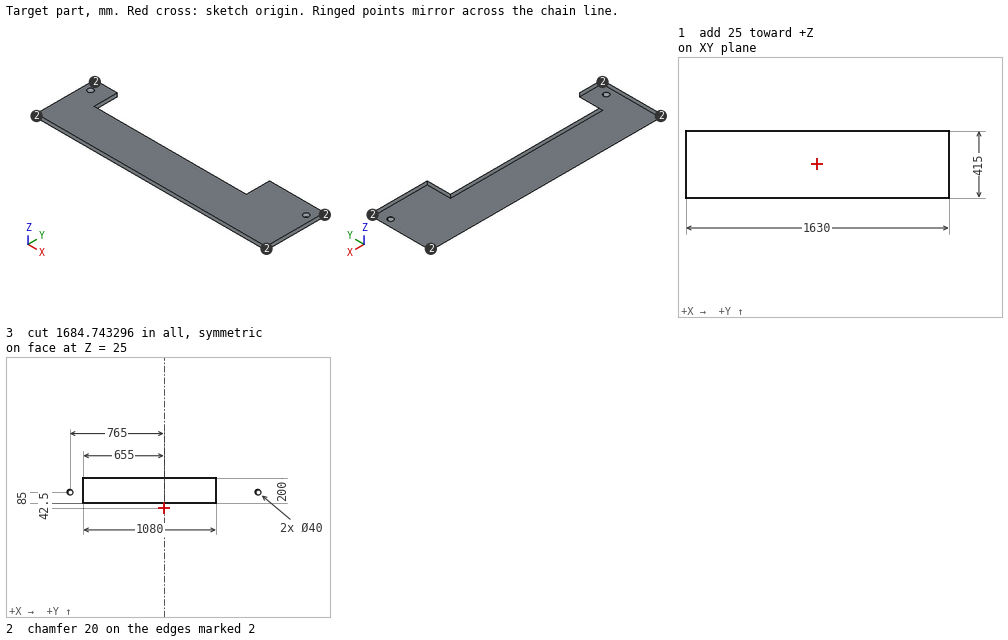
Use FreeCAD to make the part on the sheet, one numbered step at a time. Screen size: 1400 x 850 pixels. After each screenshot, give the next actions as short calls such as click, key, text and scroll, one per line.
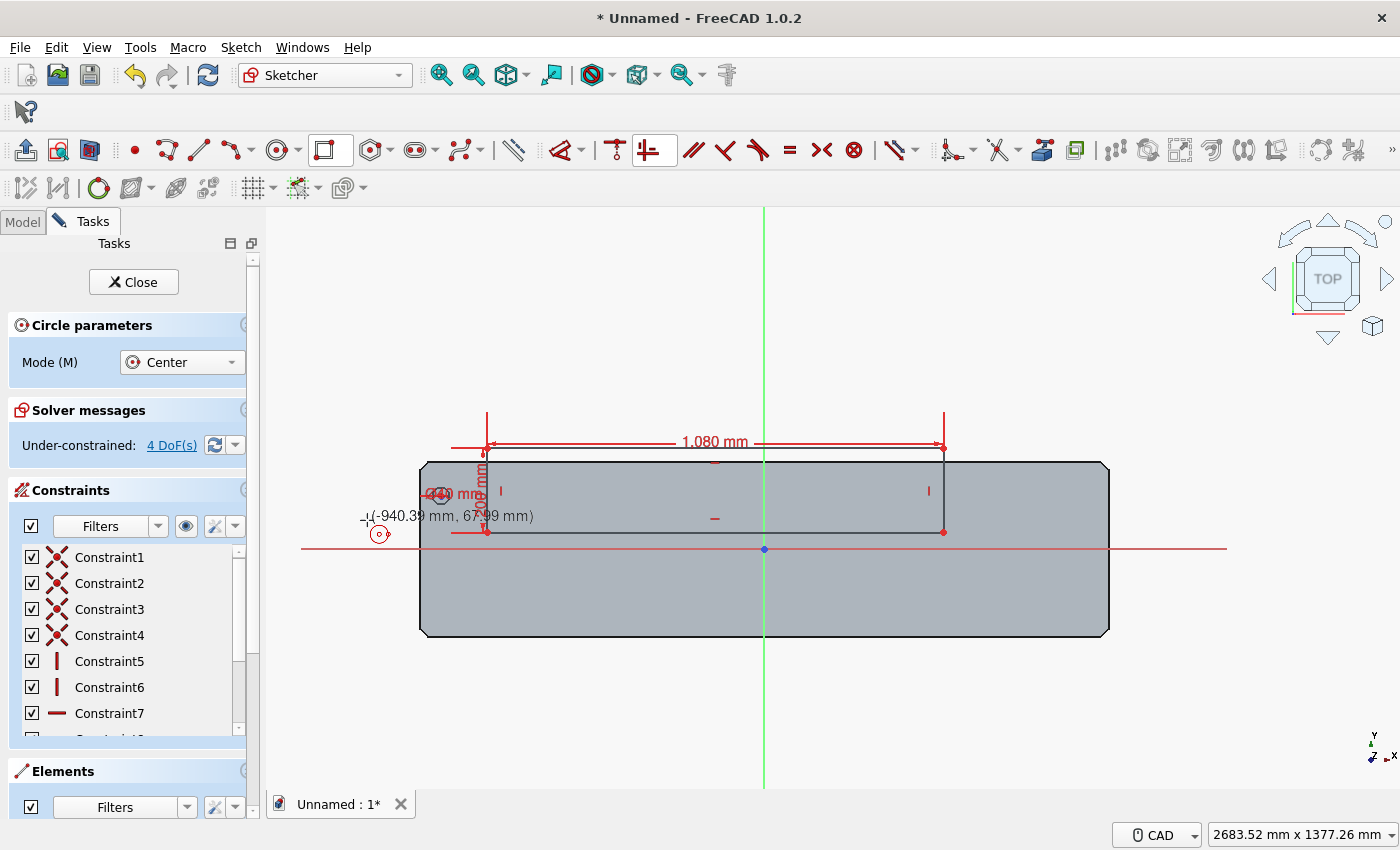
scroll(1088, 496, up, 5)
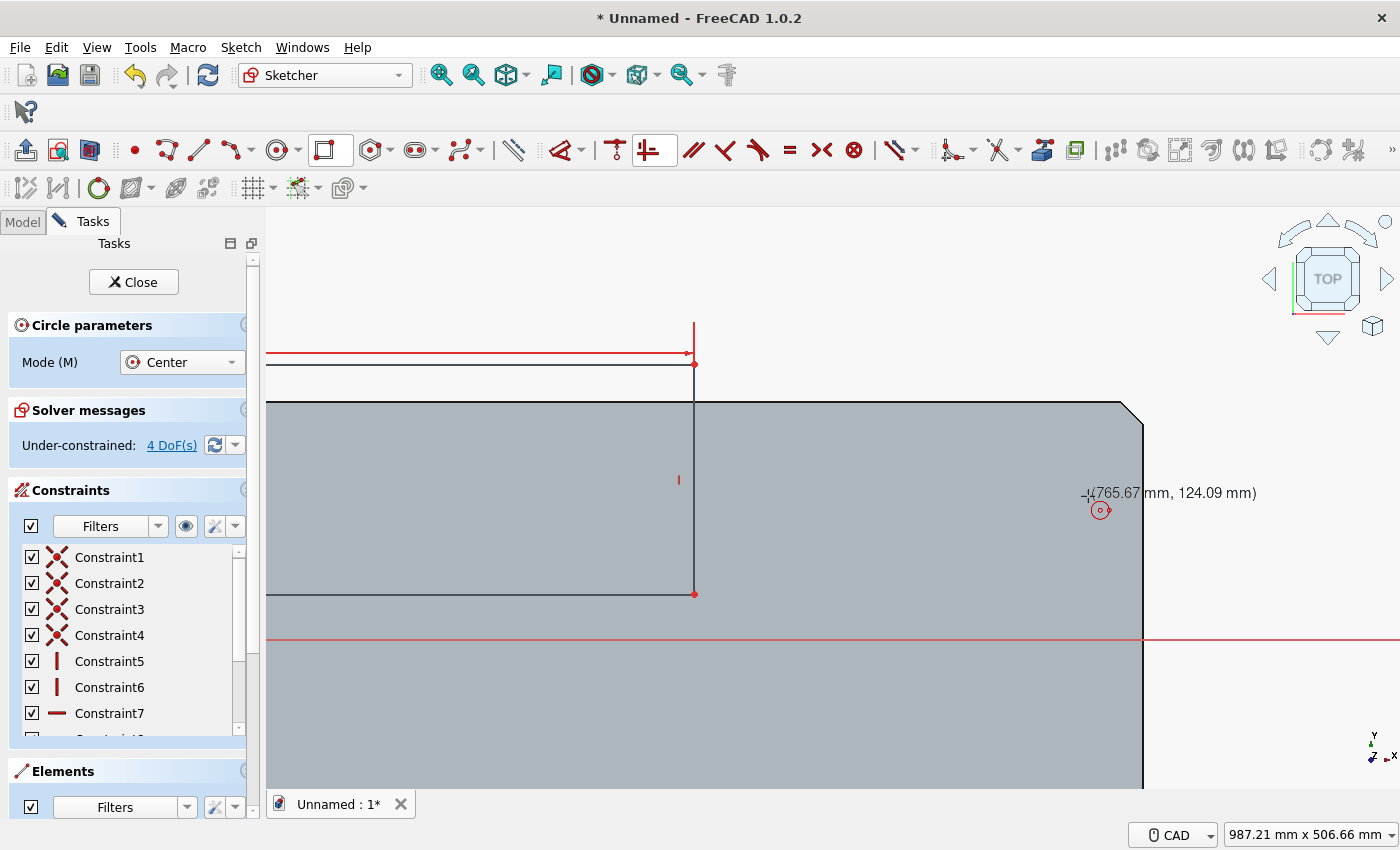
click(1086, 494)
move(1102, 478)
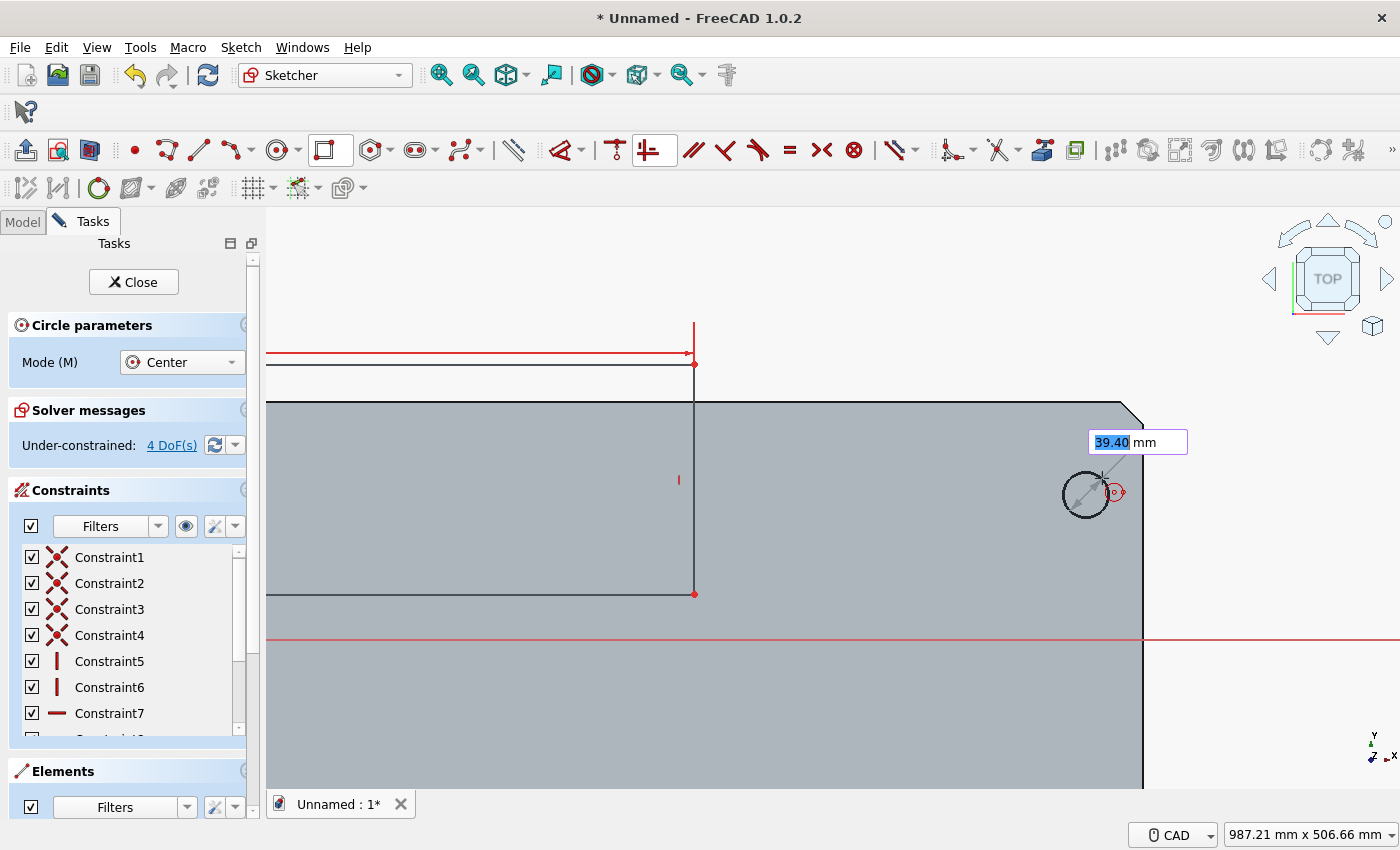
text(40)
key(Return)
key(Escape)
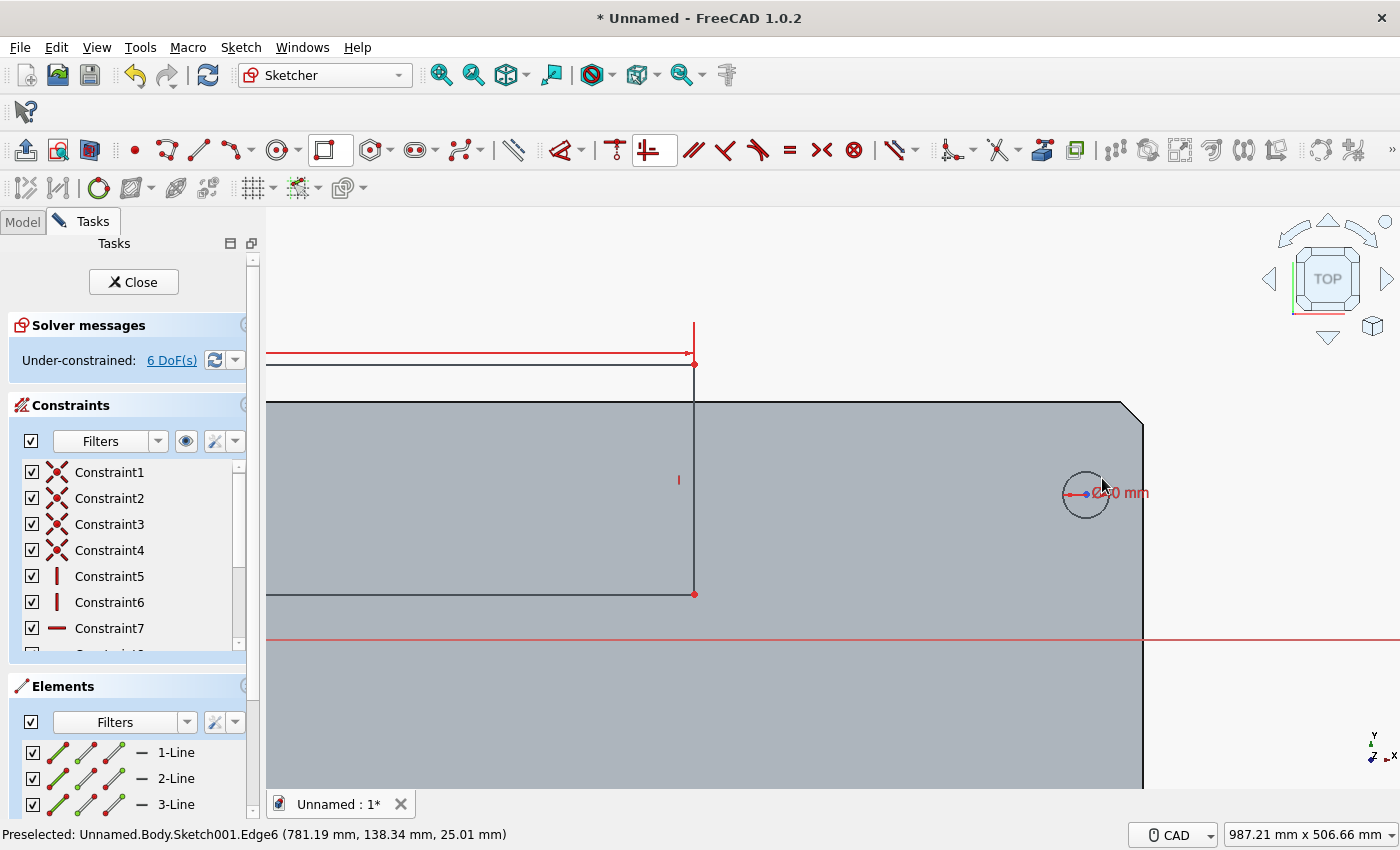
scroll(1089, 496, down, 5)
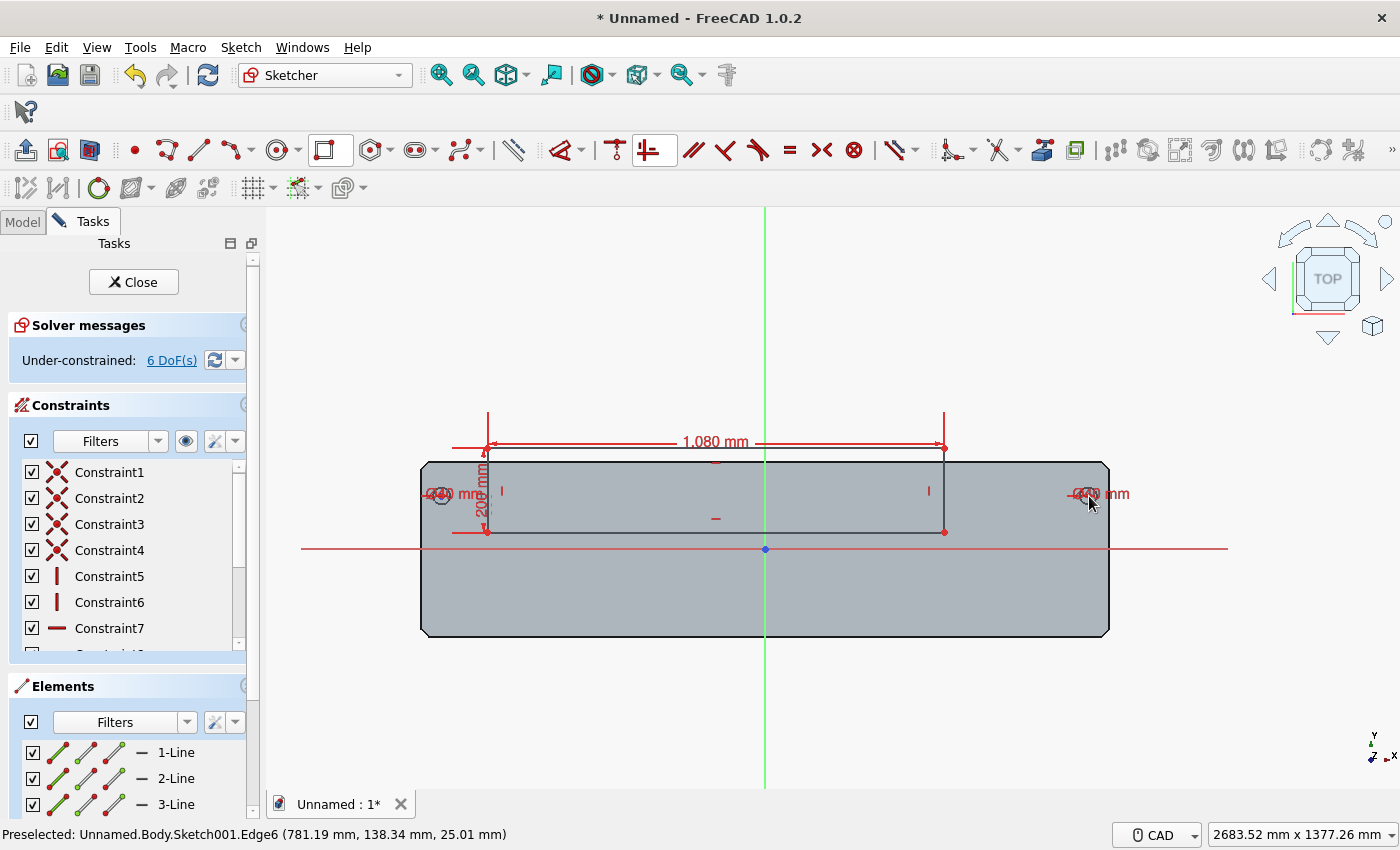
click(442, 496)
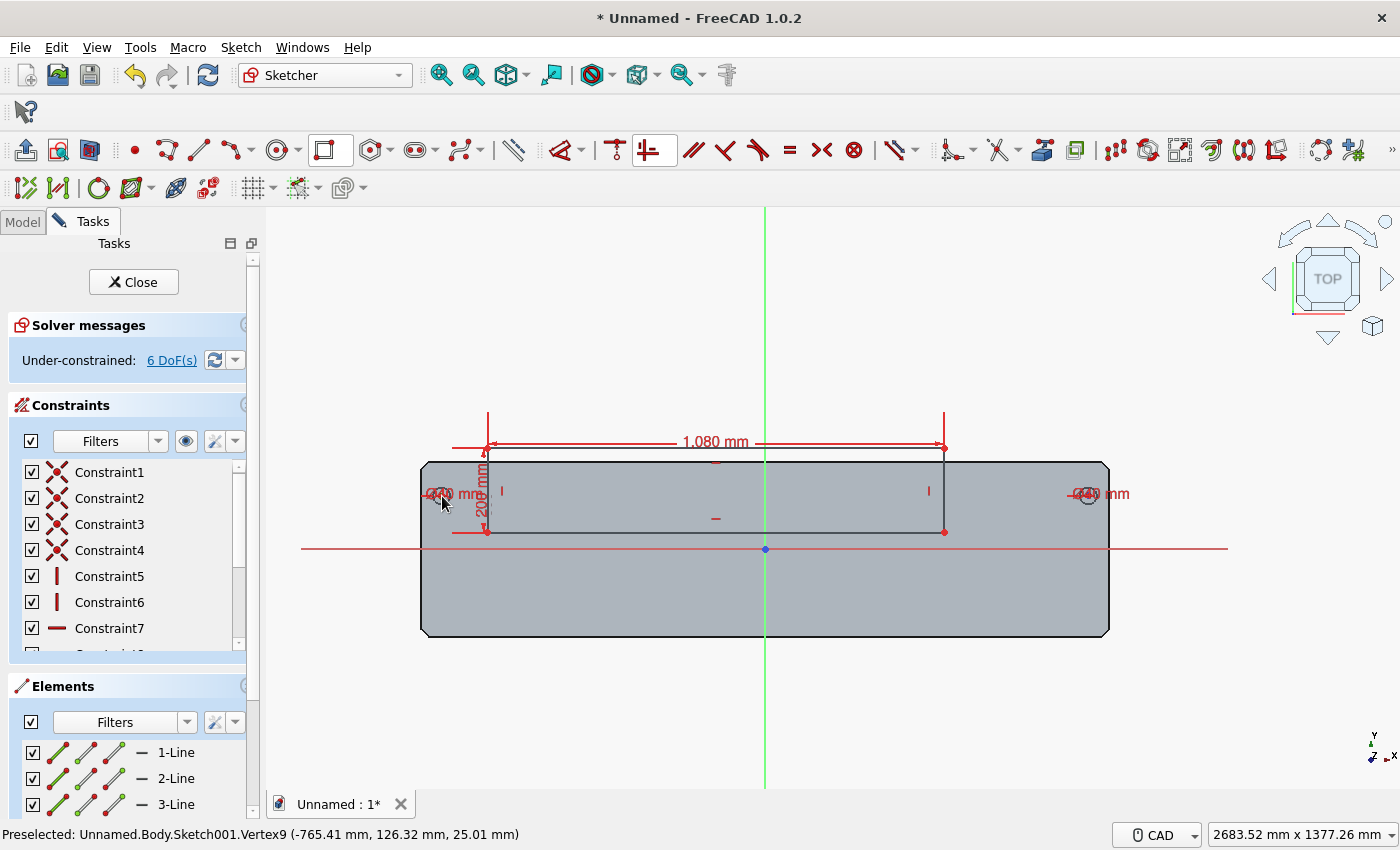
click(1088, 496)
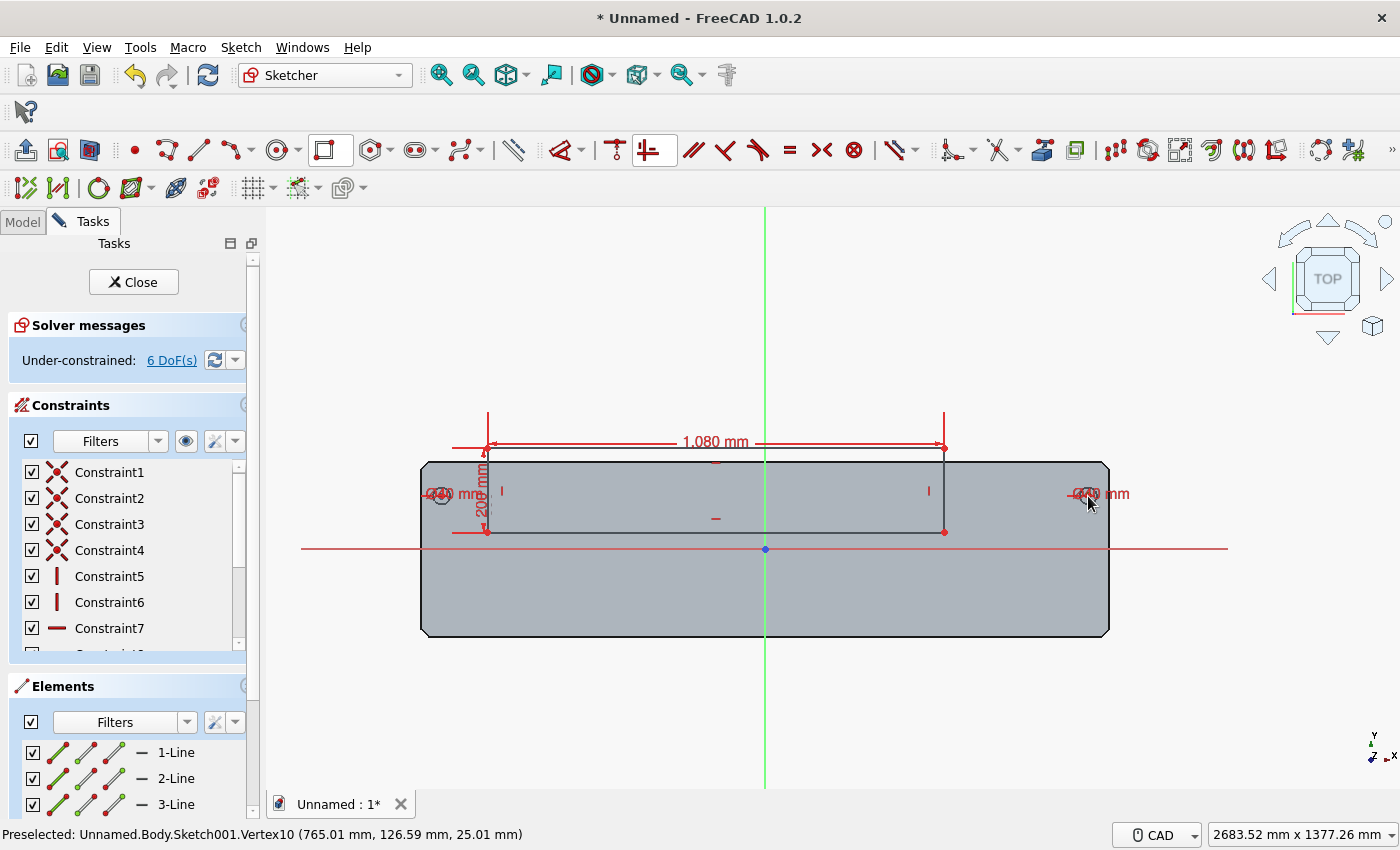
click(765, 723)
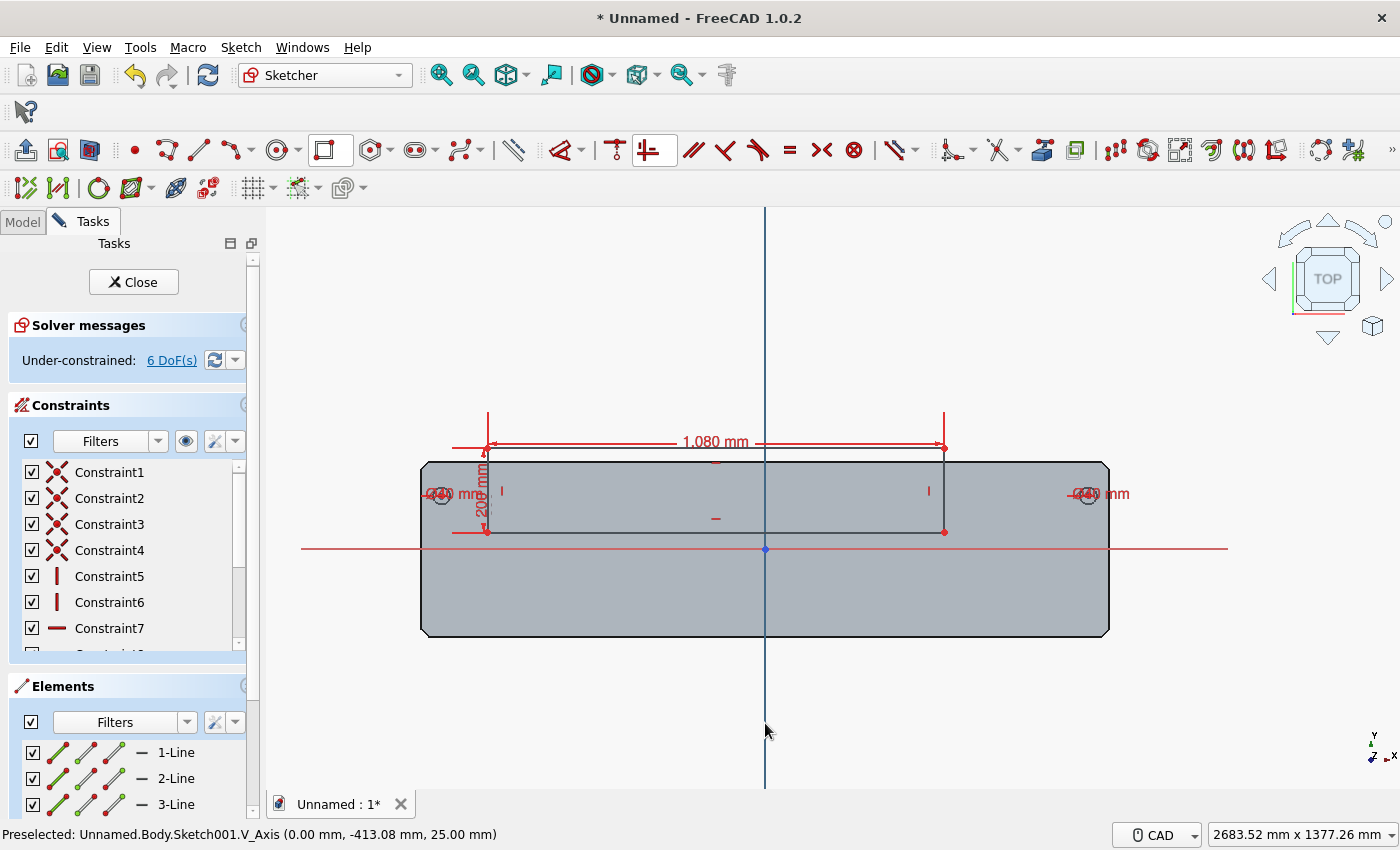
click(822, 150)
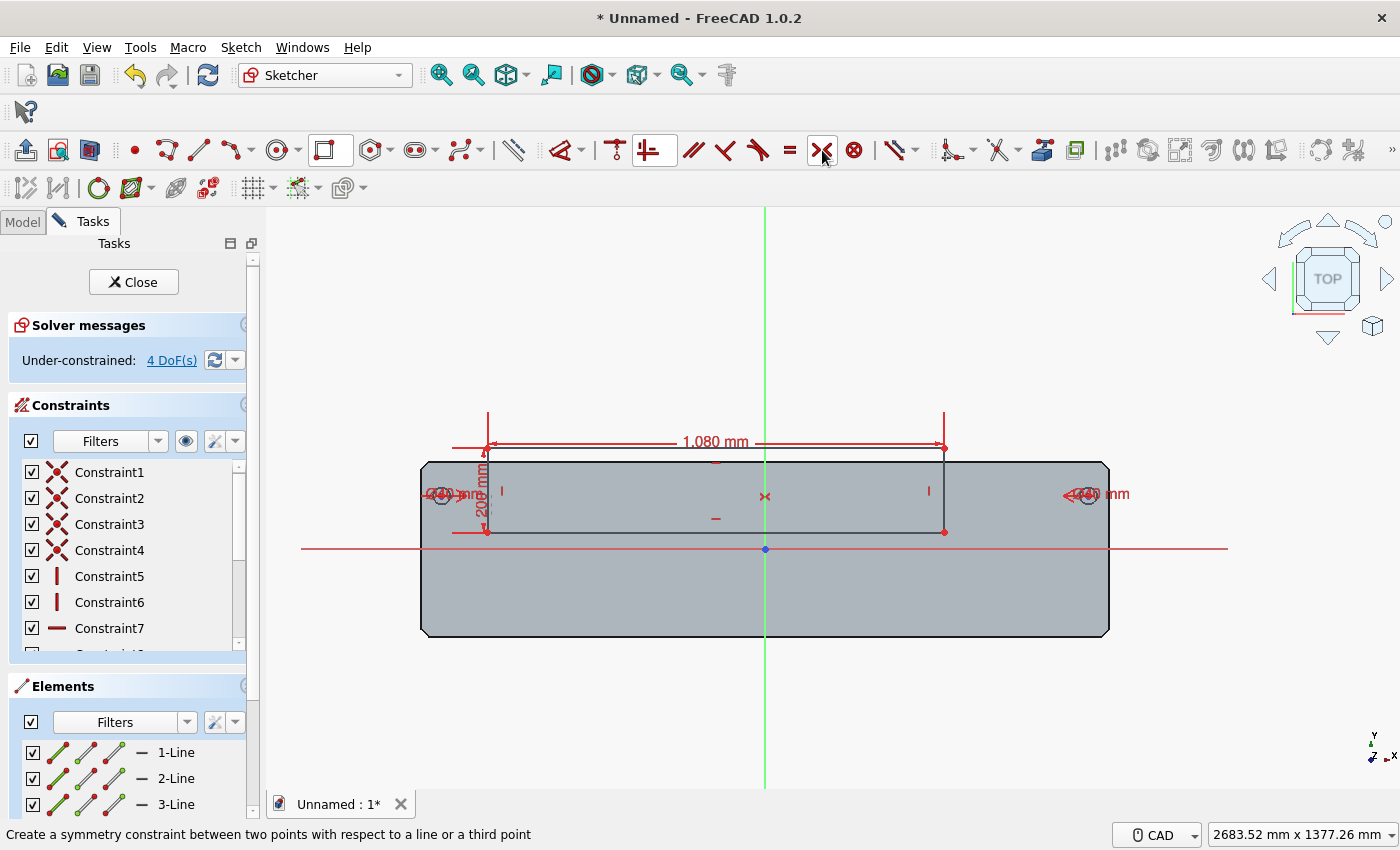
click(442, 496)